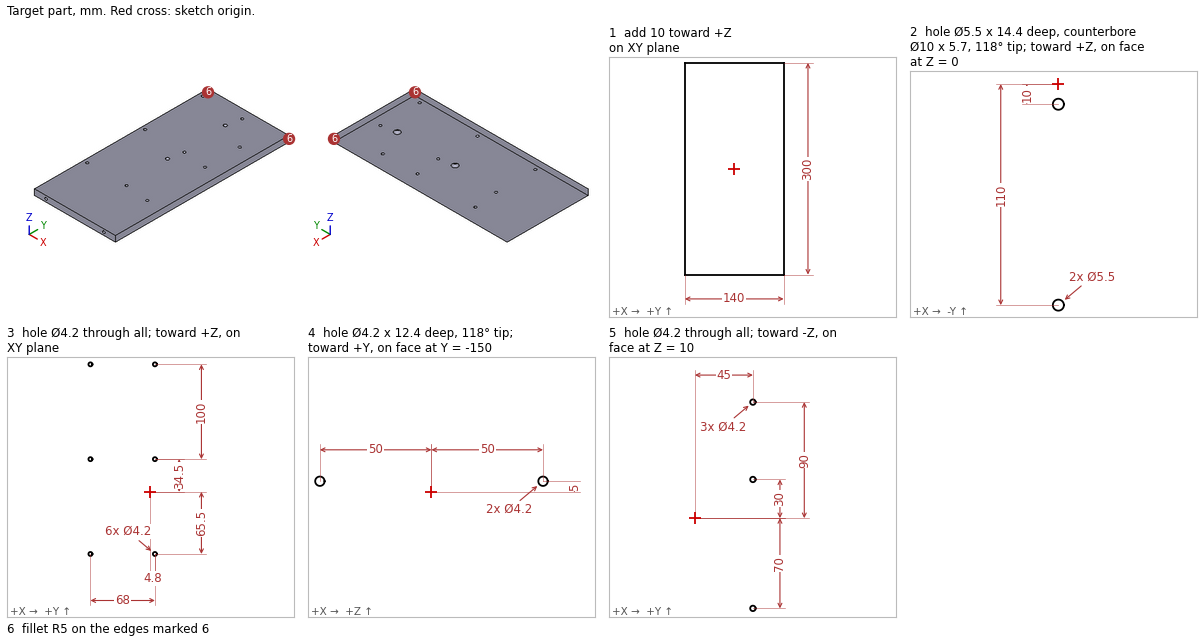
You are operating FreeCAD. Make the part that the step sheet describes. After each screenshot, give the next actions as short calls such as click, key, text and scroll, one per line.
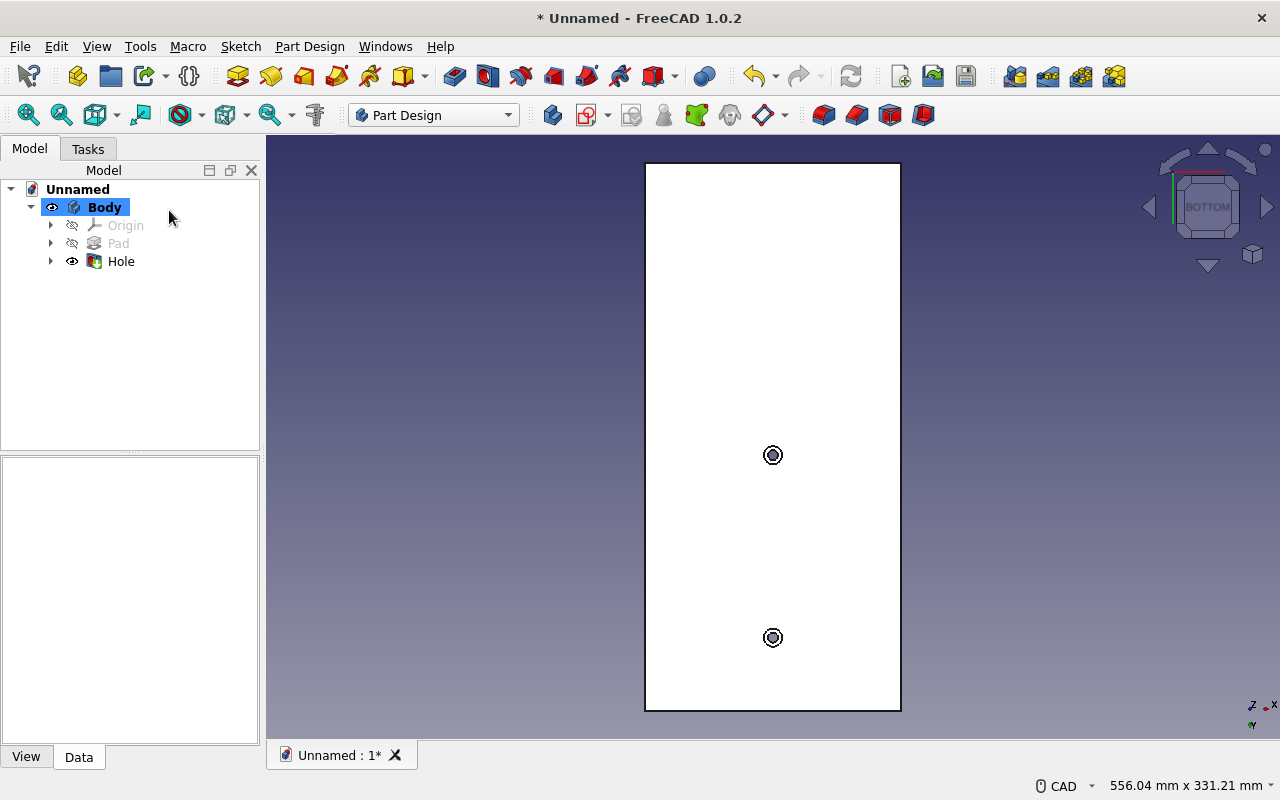
click(586, 116)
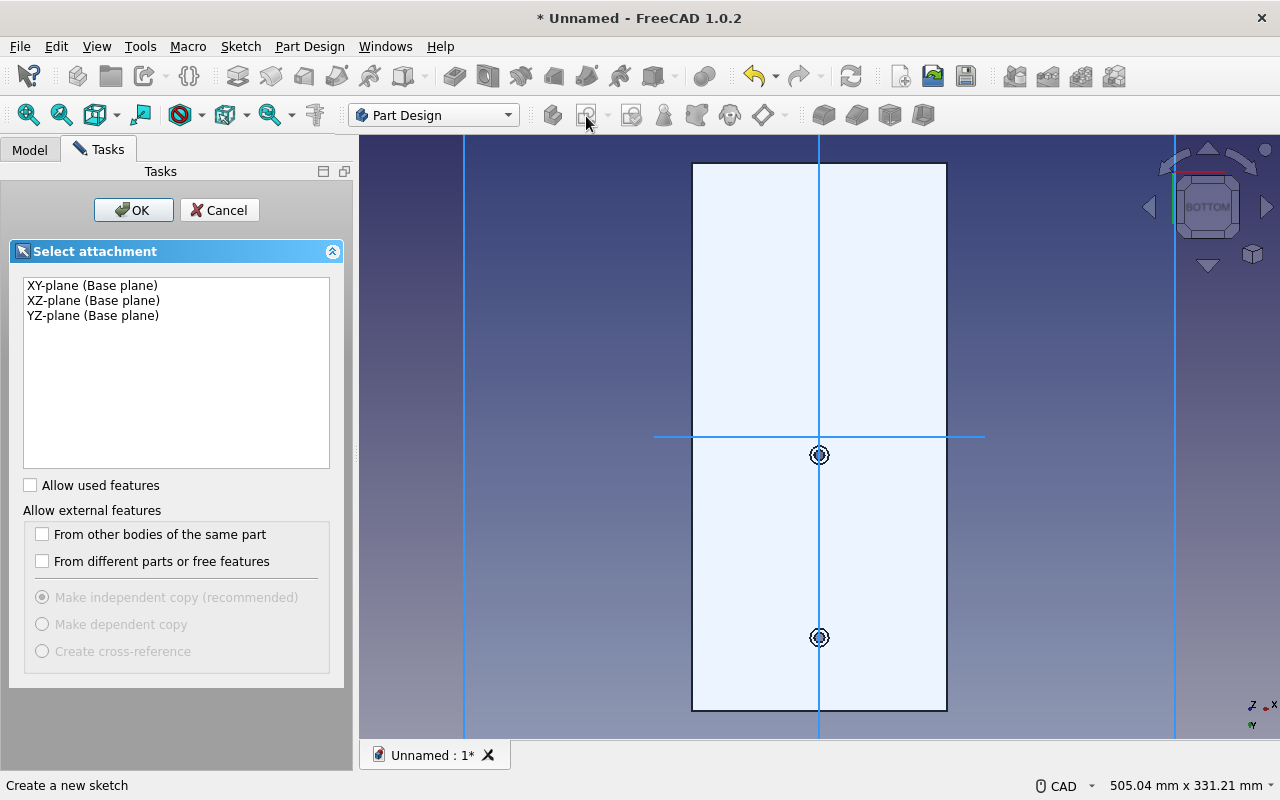
click(84, 286)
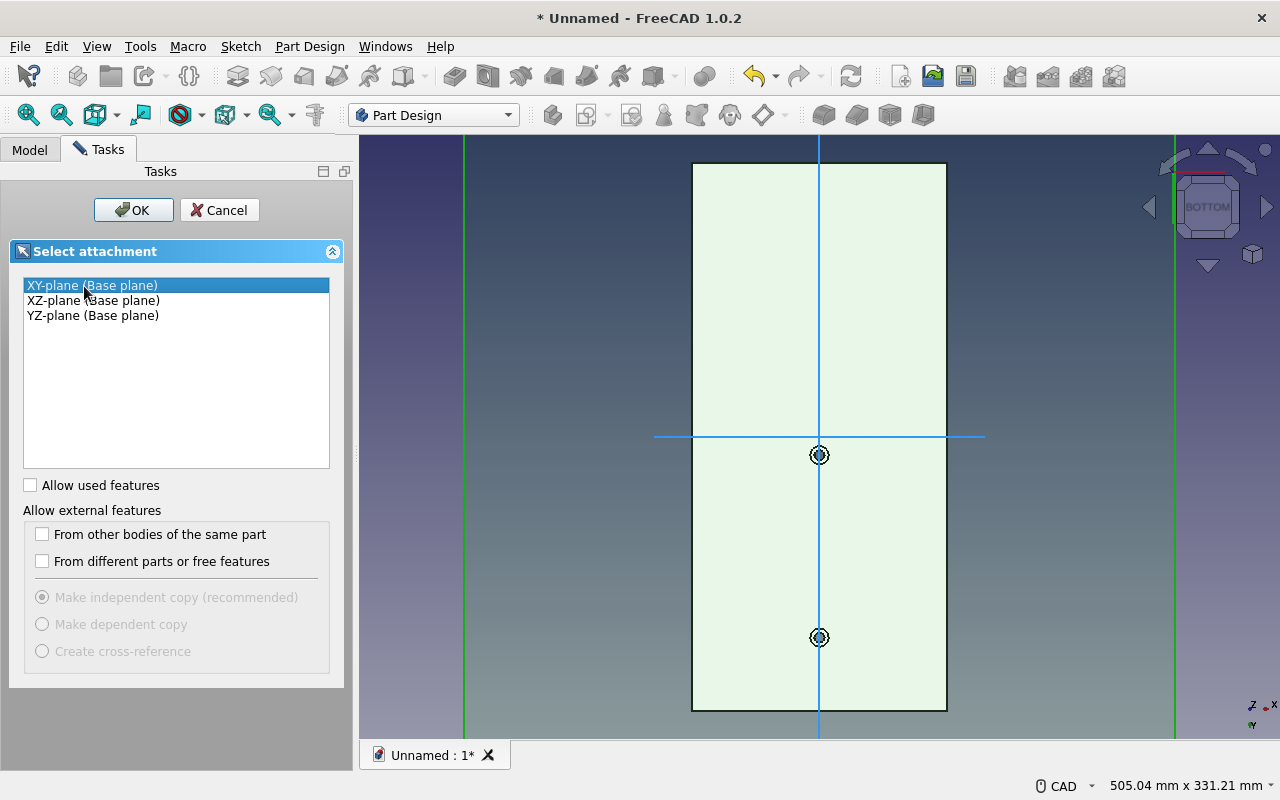
click(134, 210)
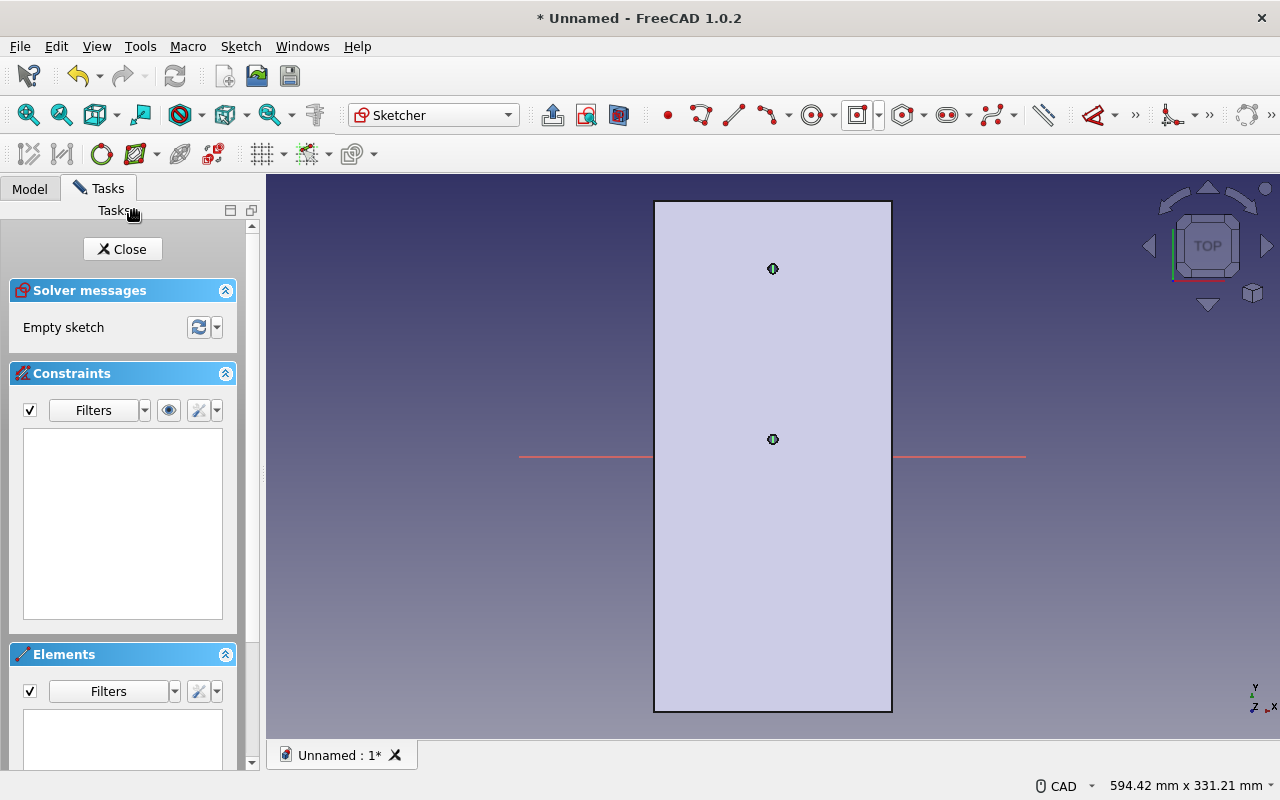
click(619, 116)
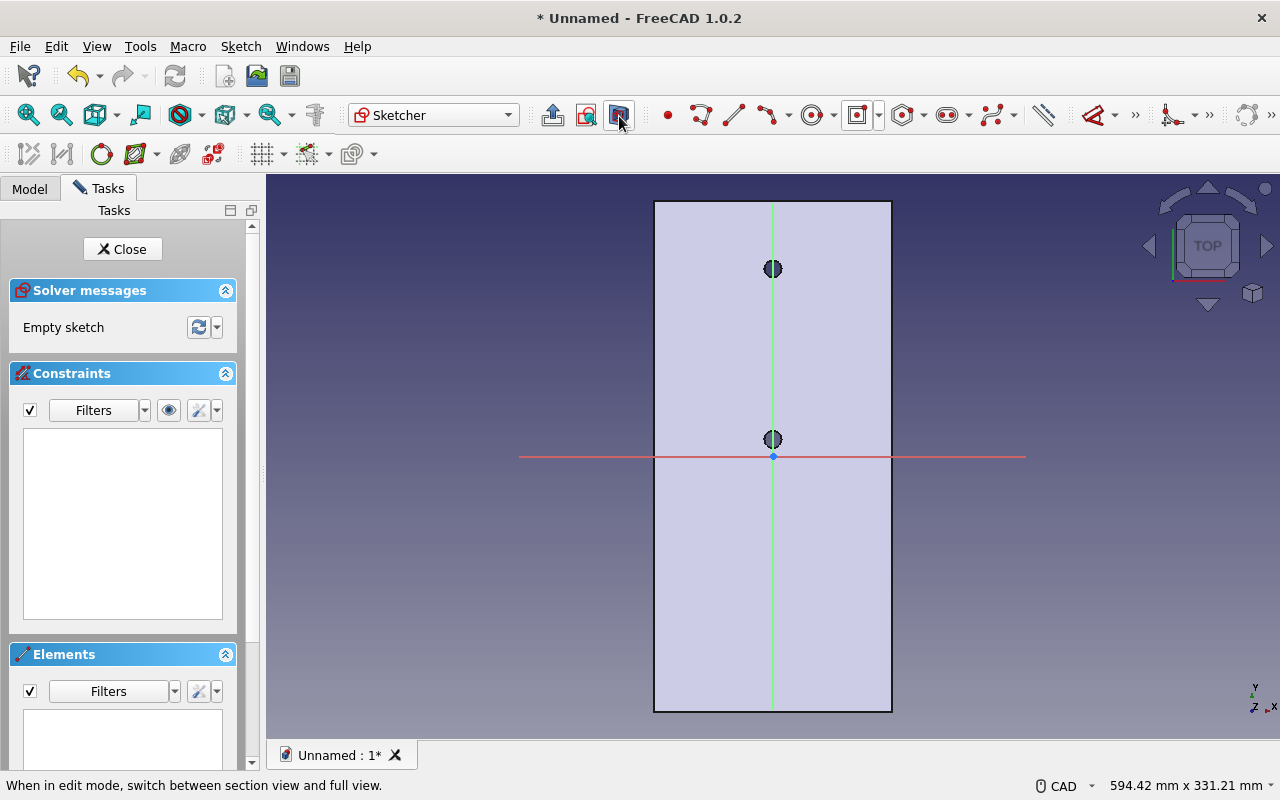
scroll(620, 711, down, 1)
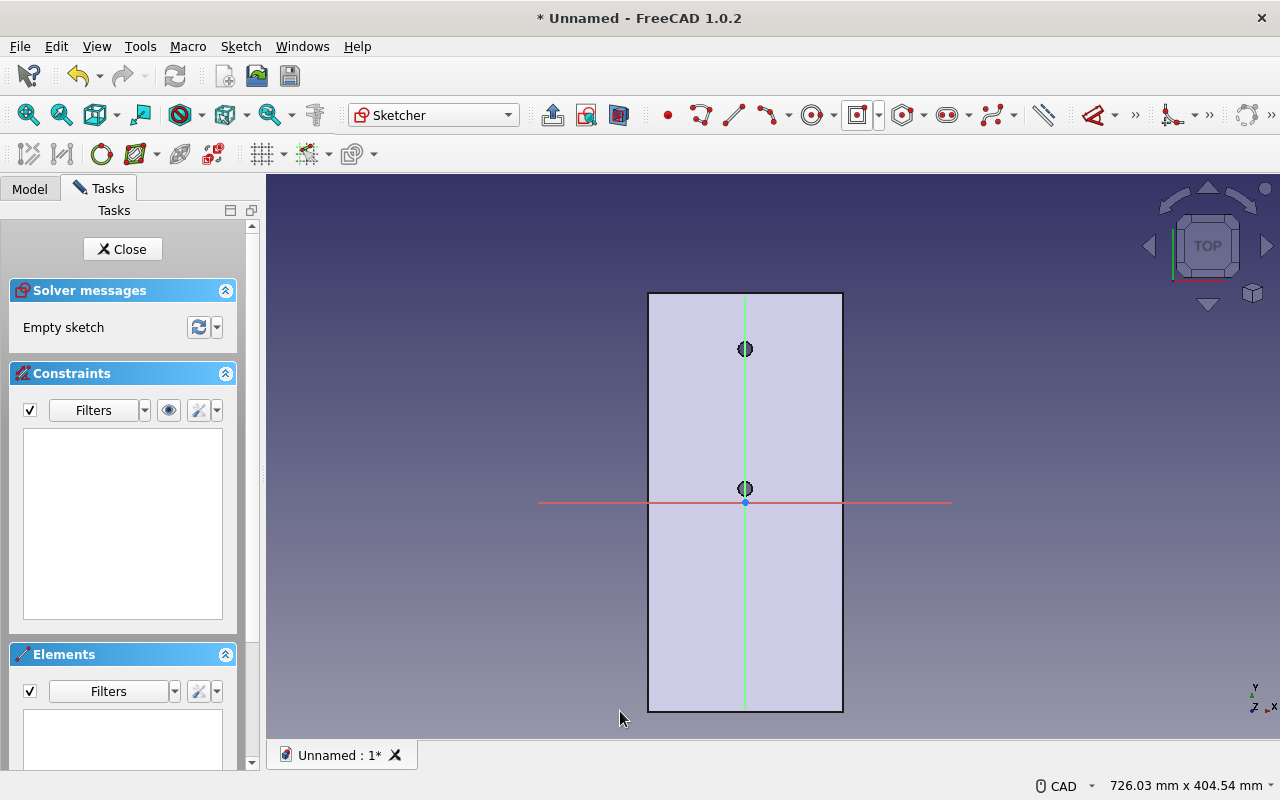
click(812, 116)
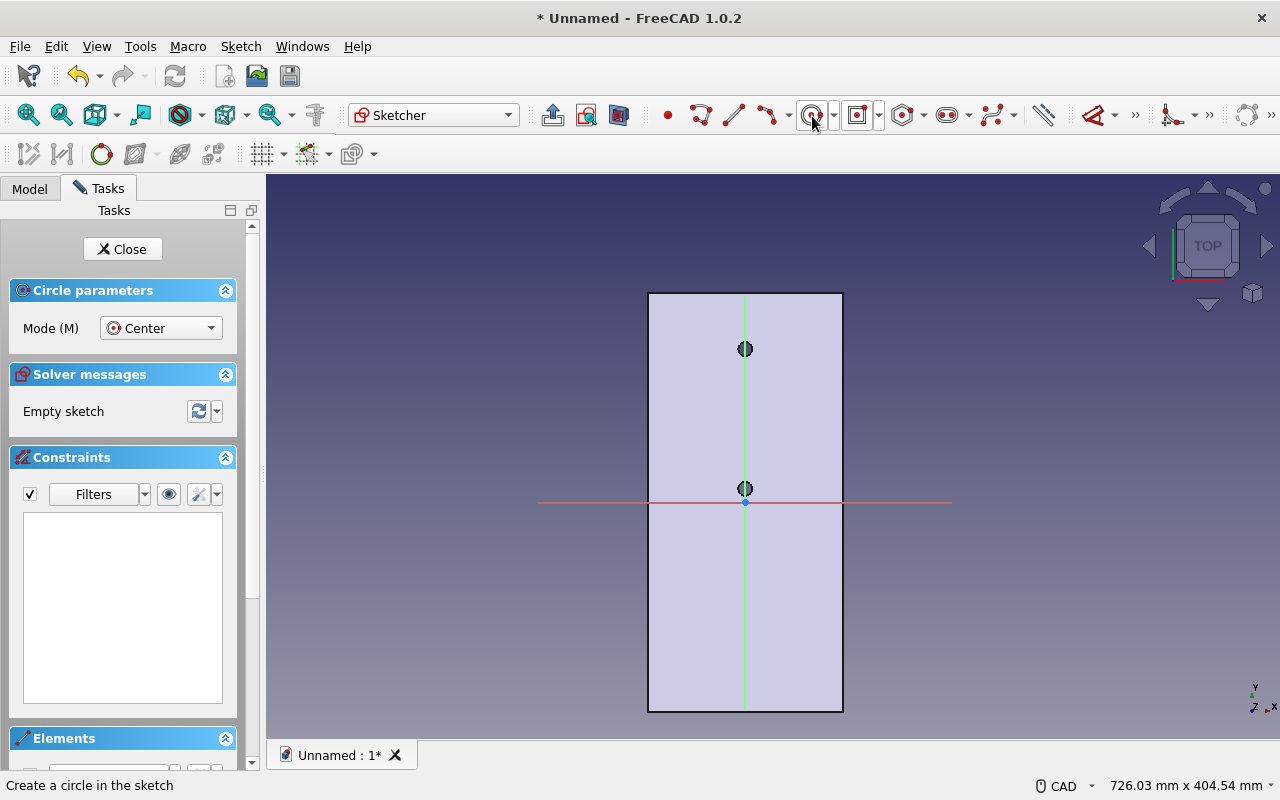
scroll(752, 594, up, 11)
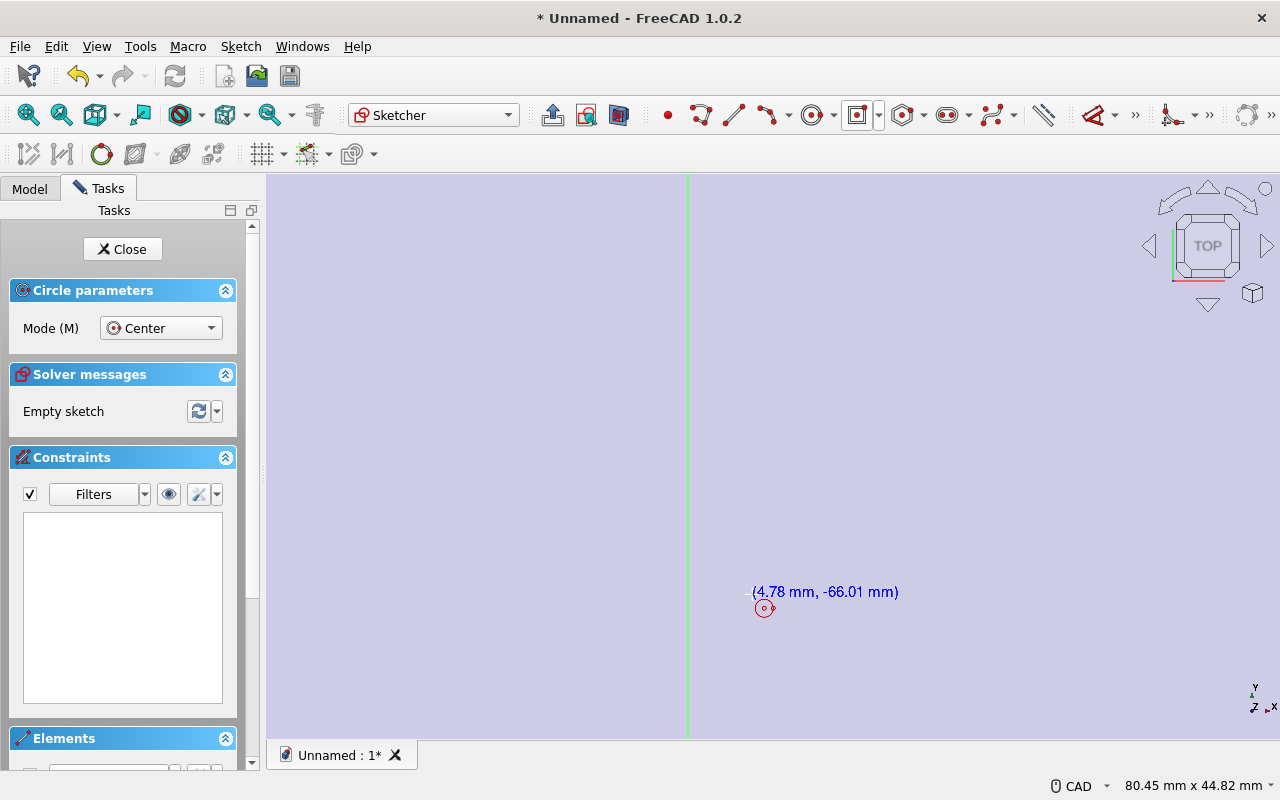
scroll(765, 633, down, 10)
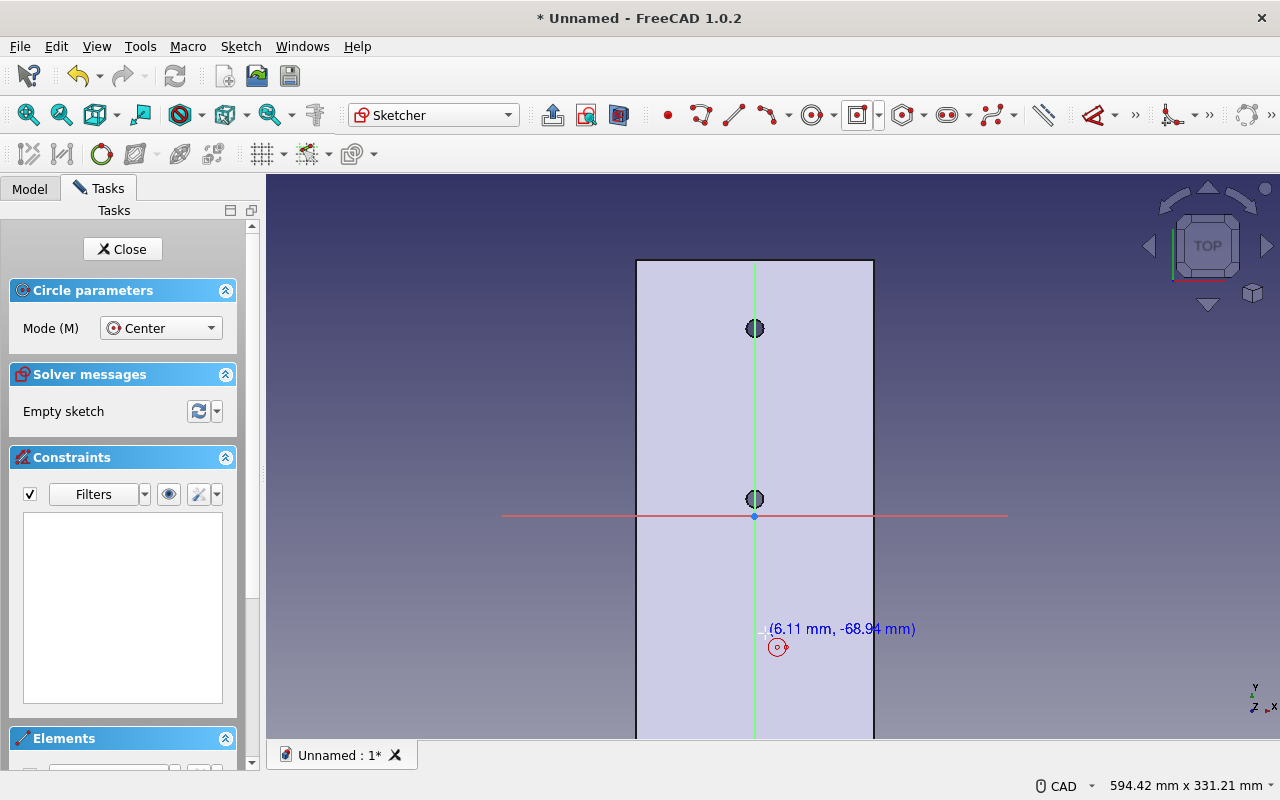
scroll(763, 628, up, 4)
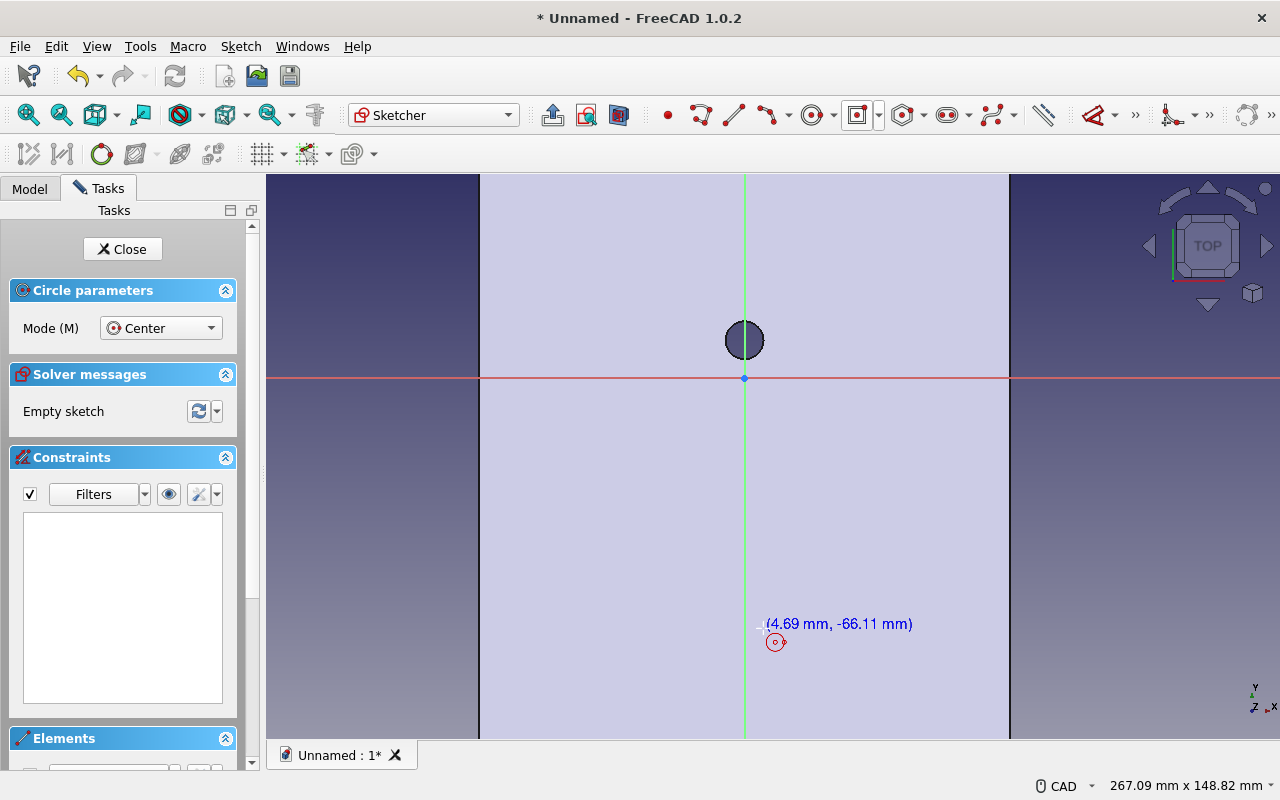
click(763, 627)